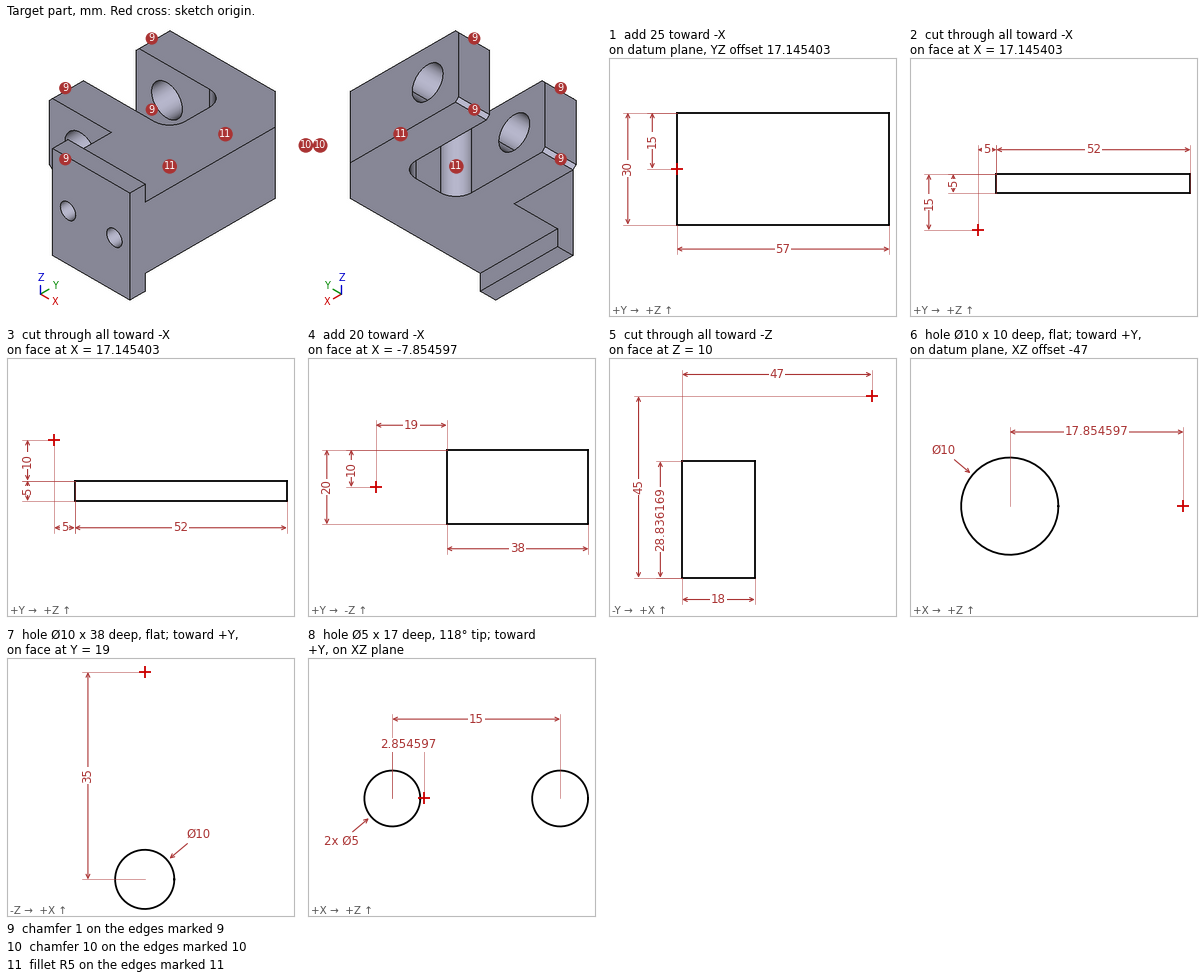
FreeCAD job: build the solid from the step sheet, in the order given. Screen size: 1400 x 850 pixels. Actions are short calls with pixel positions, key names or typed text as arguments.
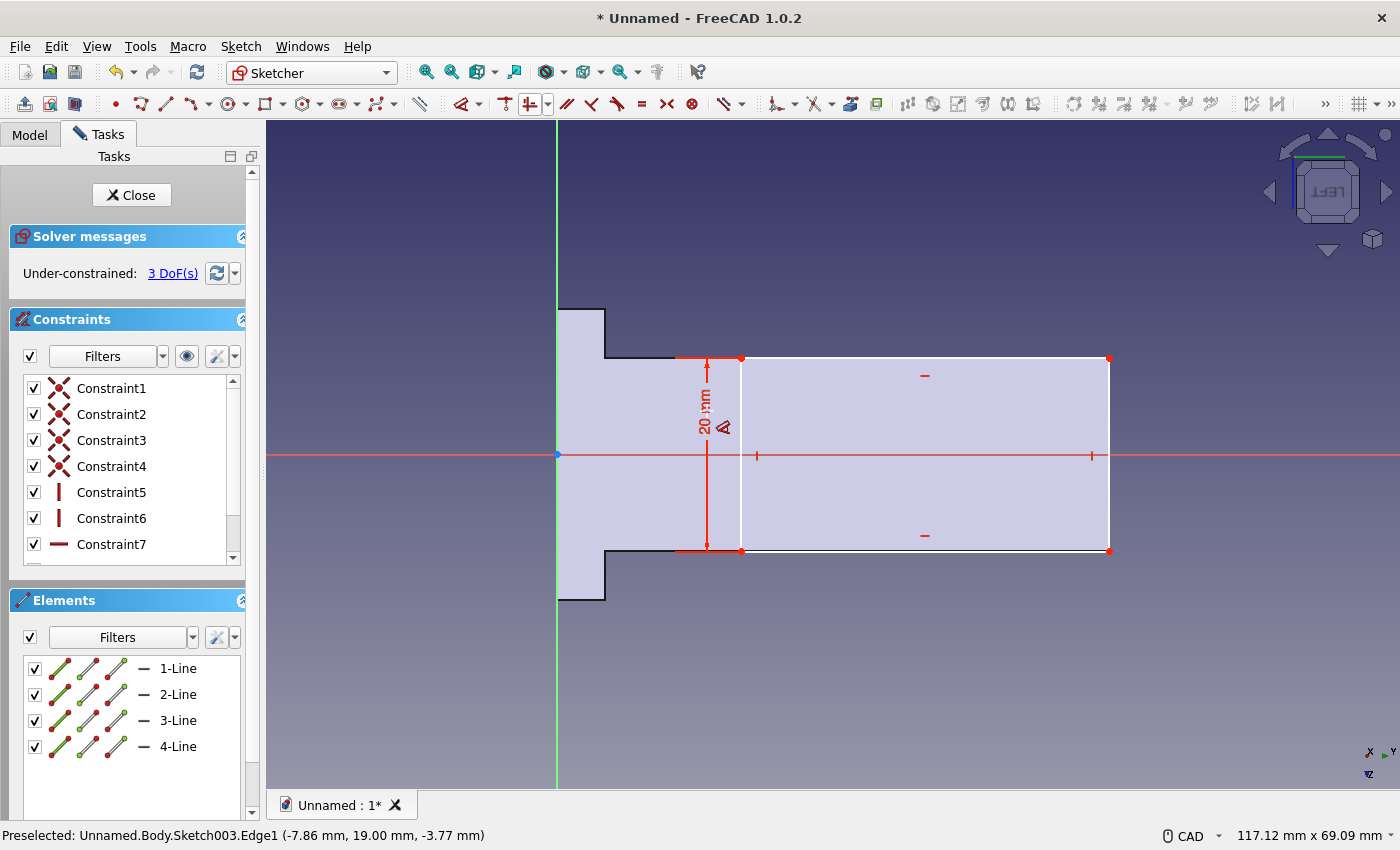
click(851, 552)
click(925, 586)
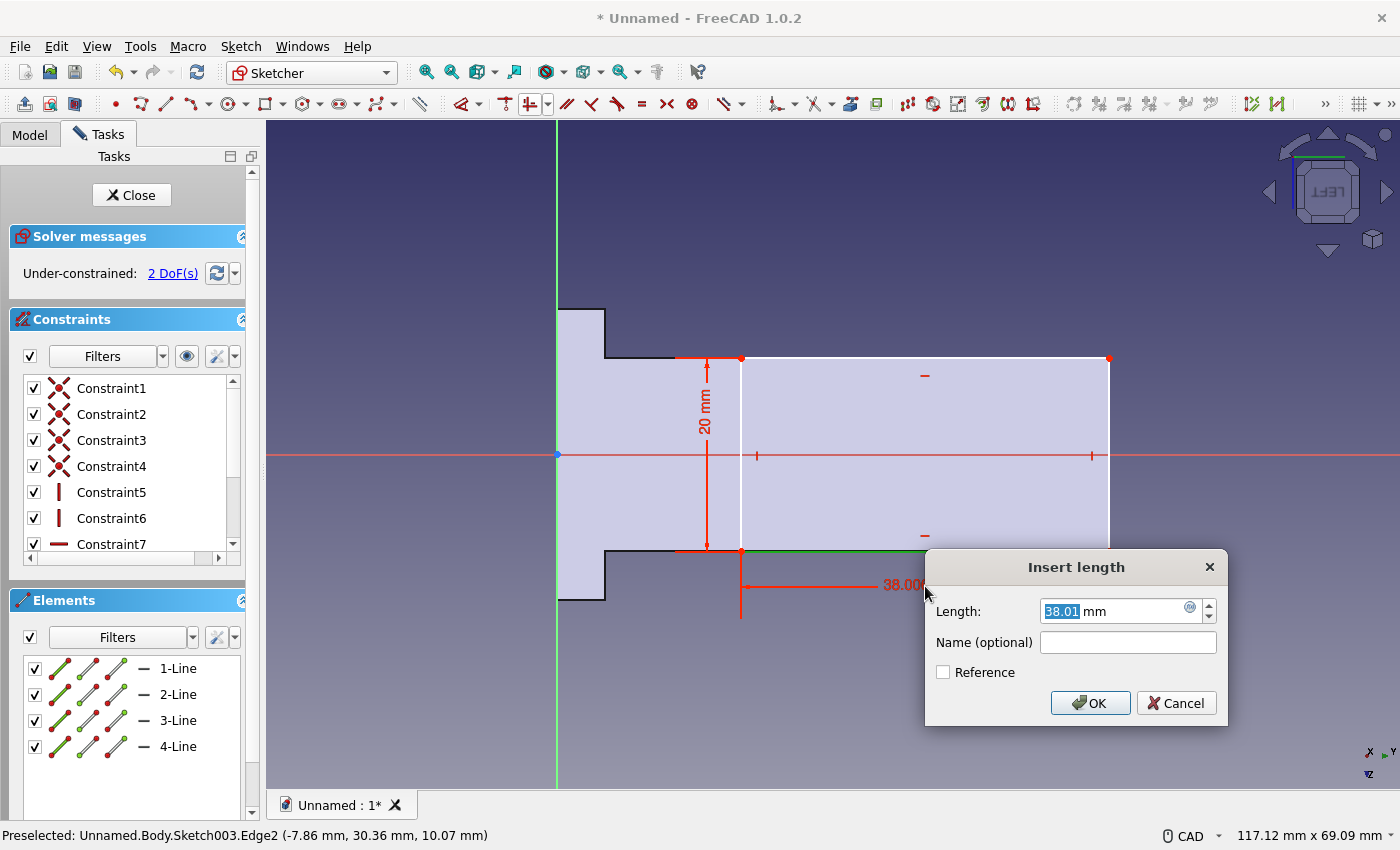
text(38)
key(Return)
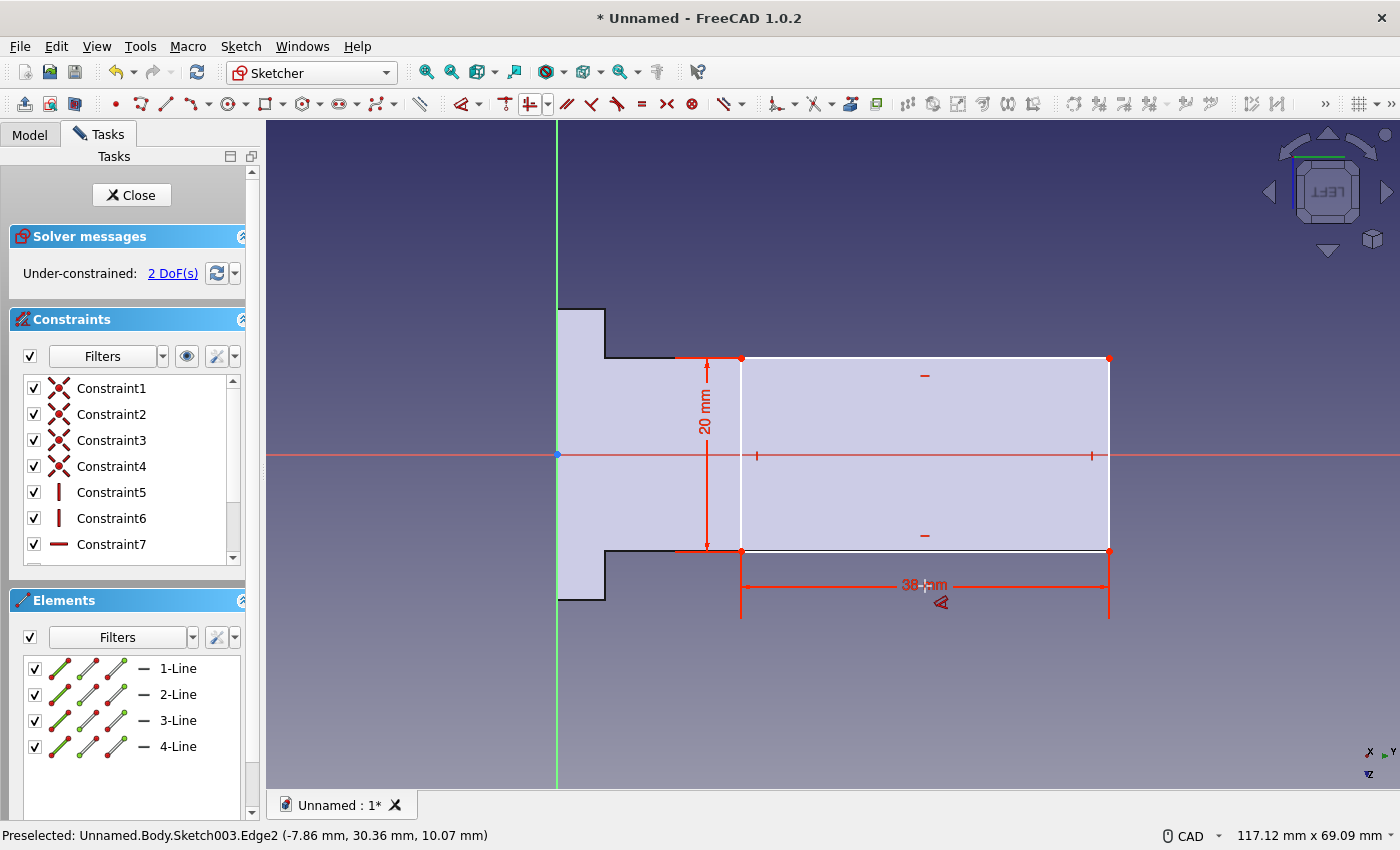
click(741, 358)
click(649, 324)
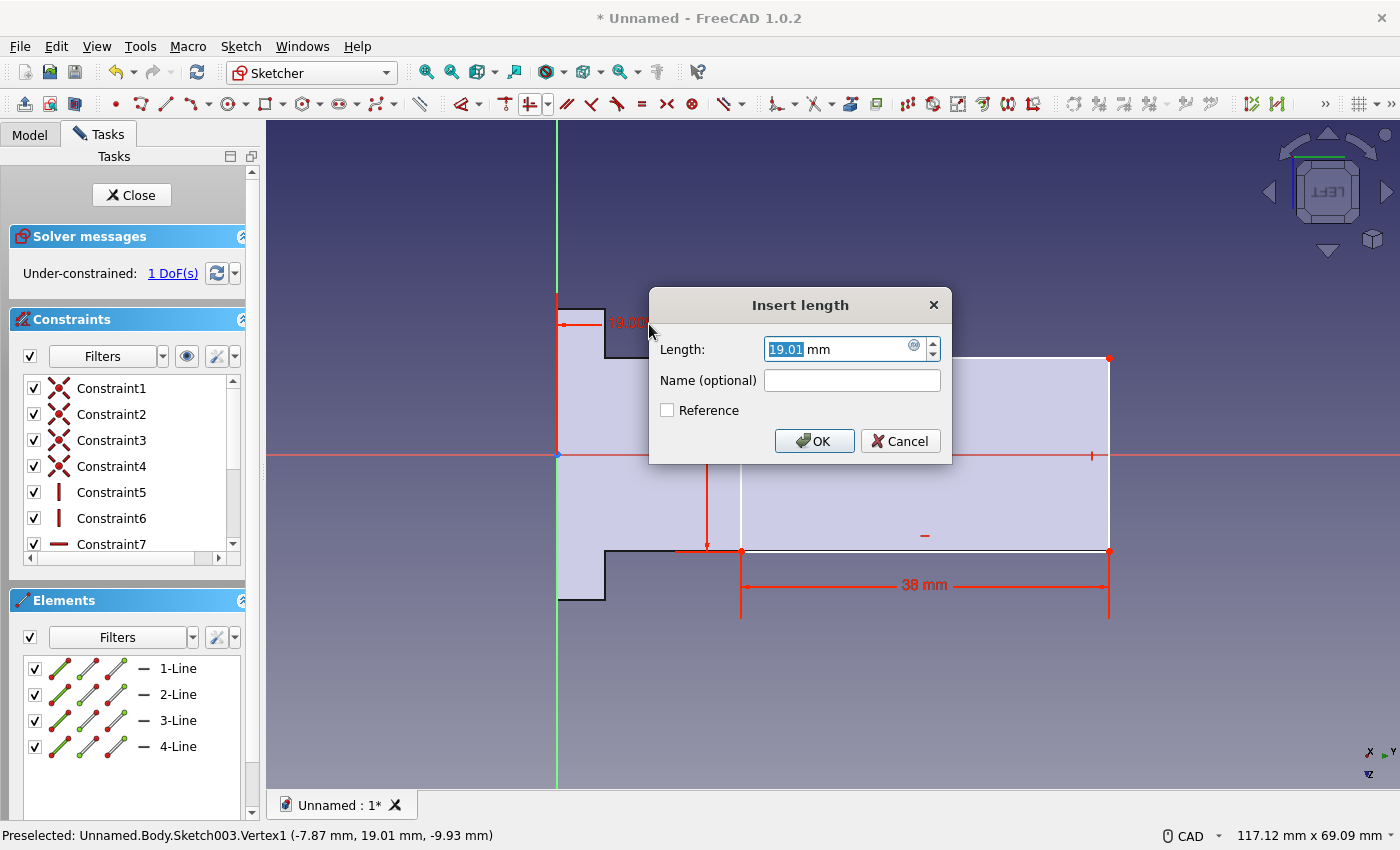
text(19)
key(Return)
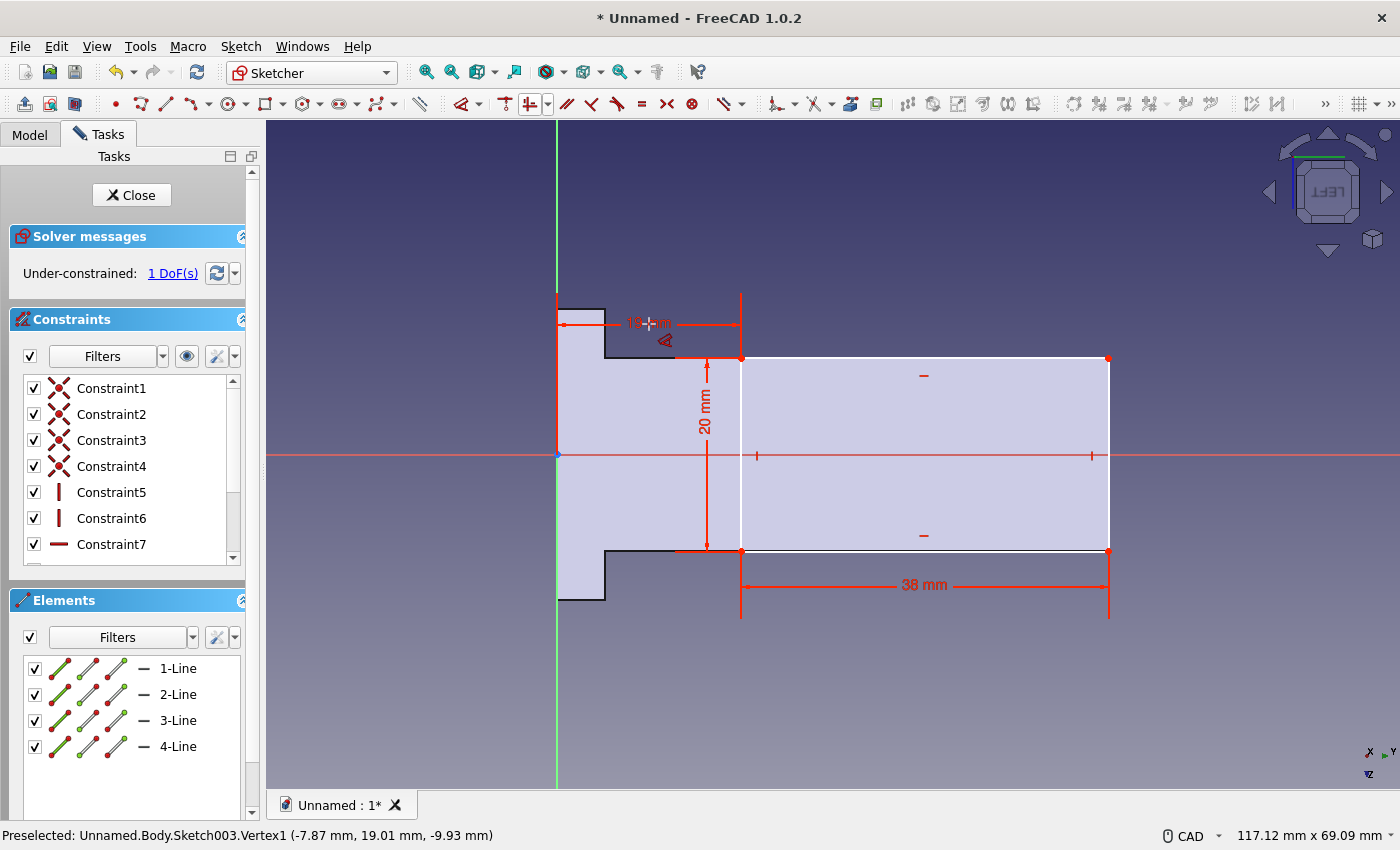
click(741, 358)
click(523, 406)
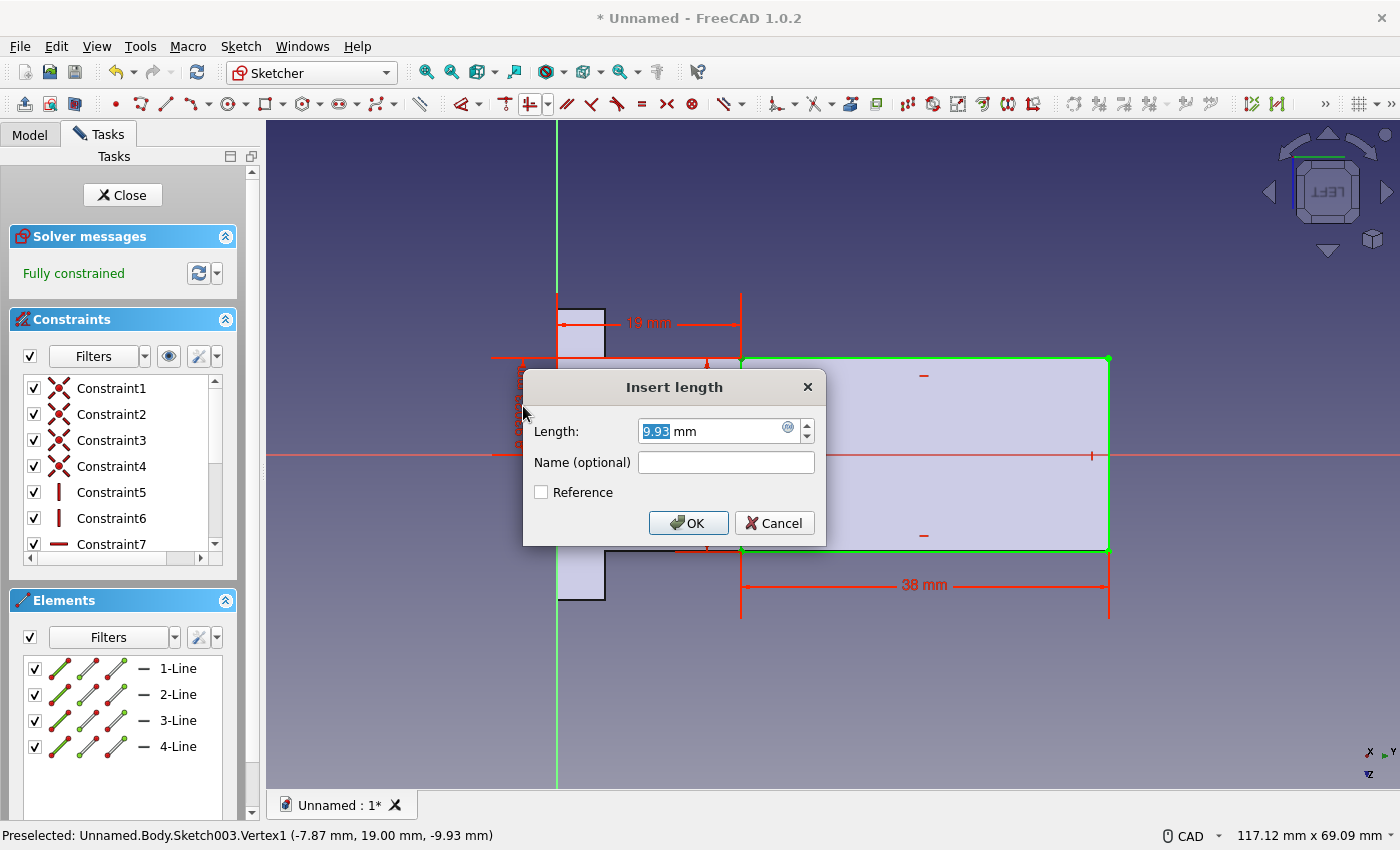
text(10)
key(Return)
key(Escape)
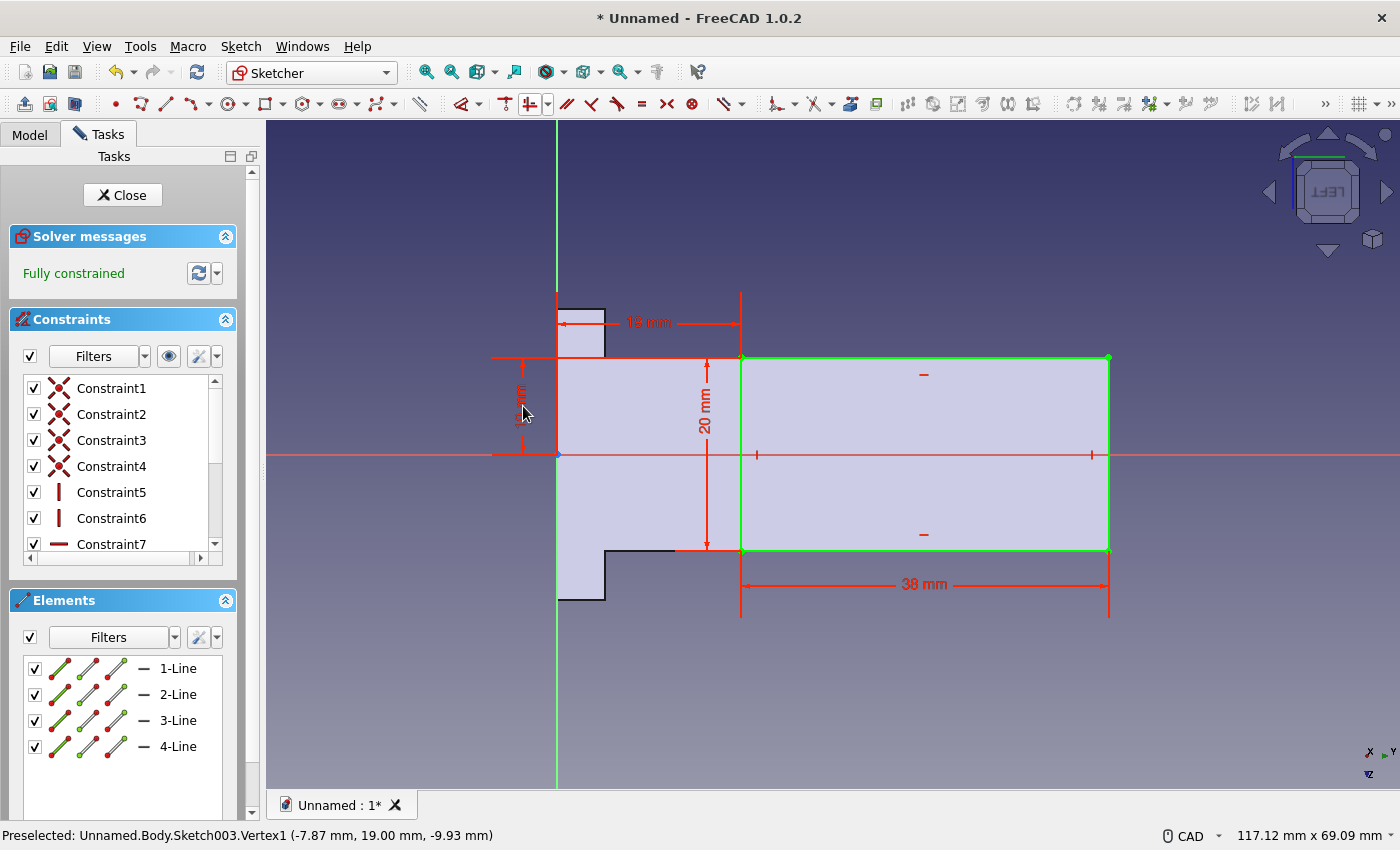
click(123, 195)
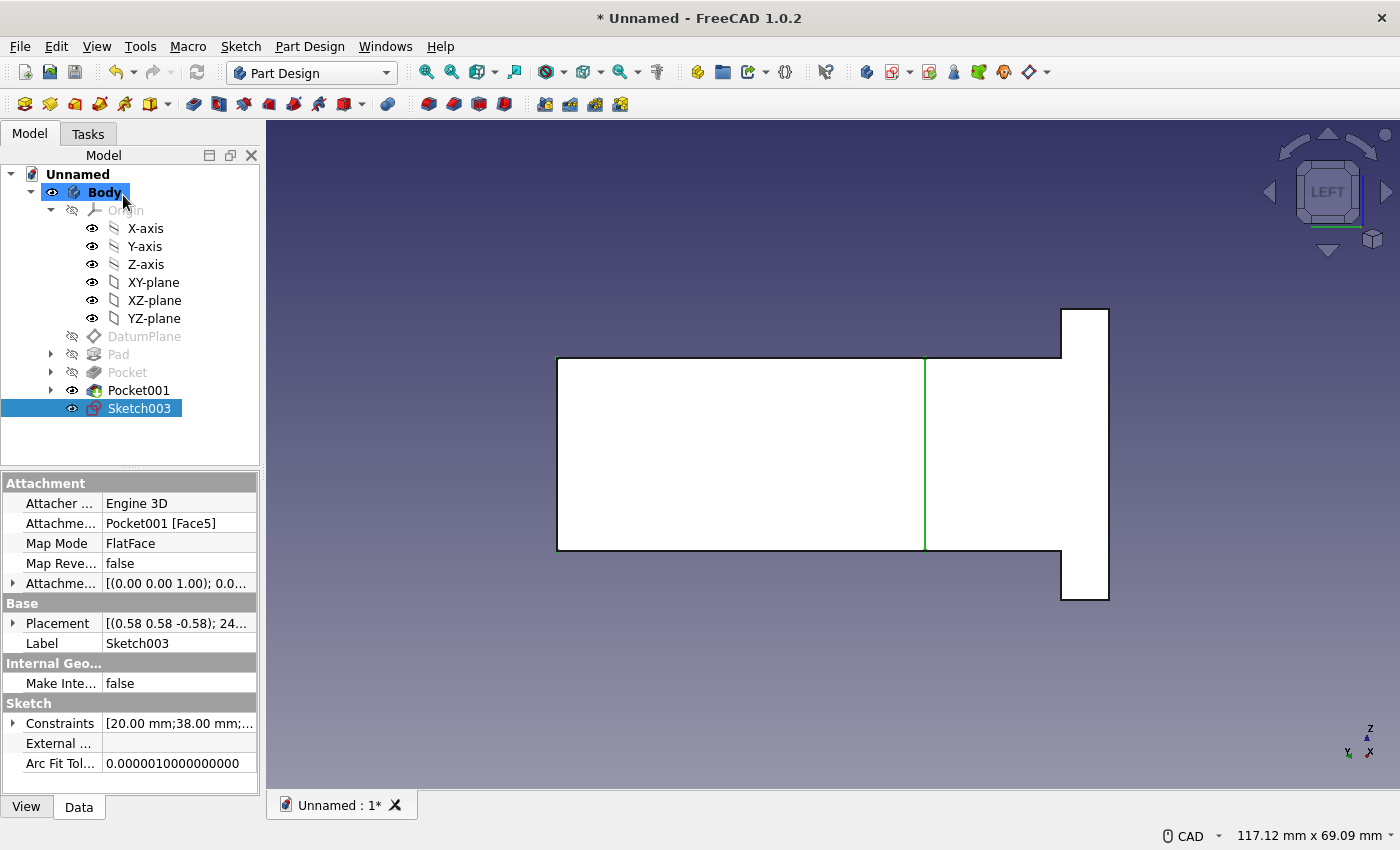
click(25, 104)